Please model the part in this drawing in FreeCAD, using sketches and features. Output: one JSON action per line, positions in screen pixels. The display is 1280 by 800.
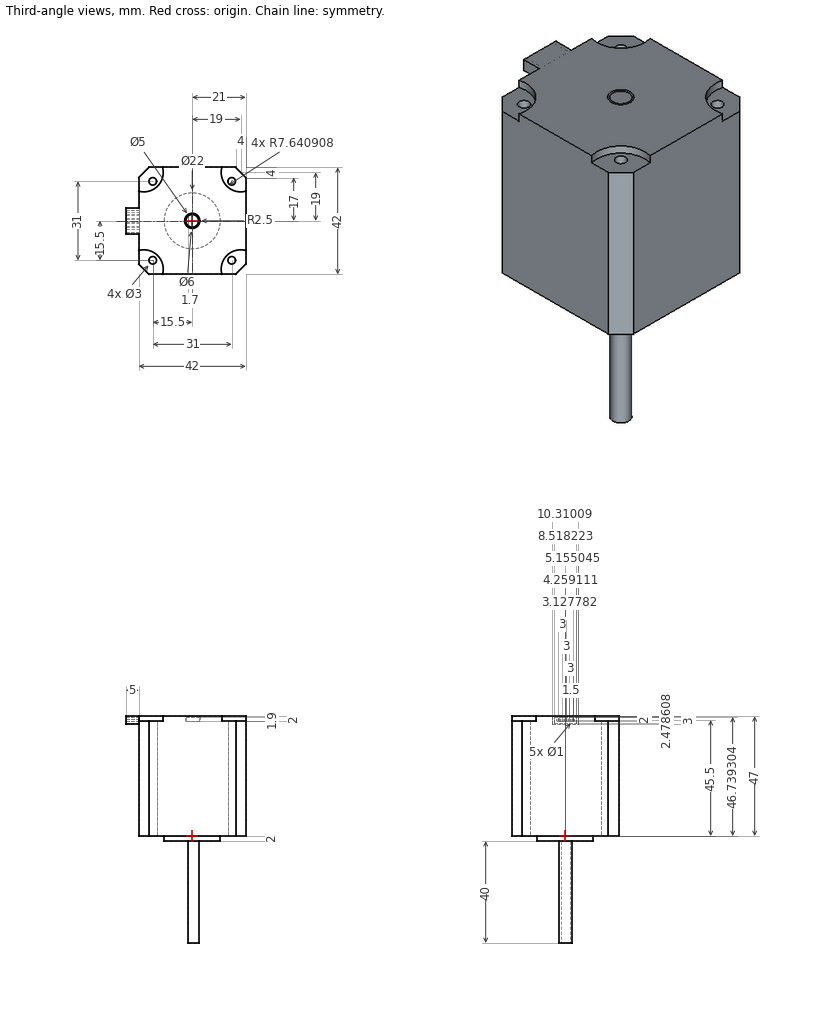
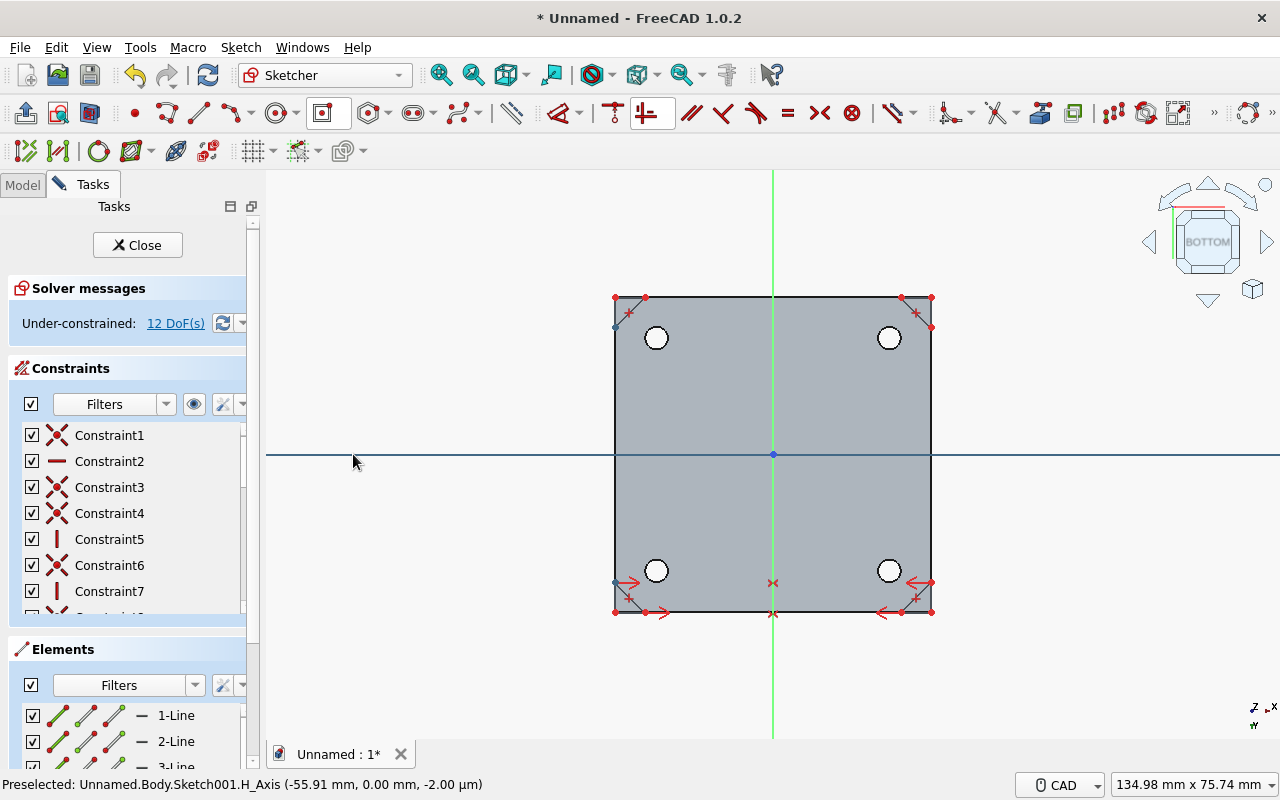
{"action": "left_click", "coordinate": [820, 114]}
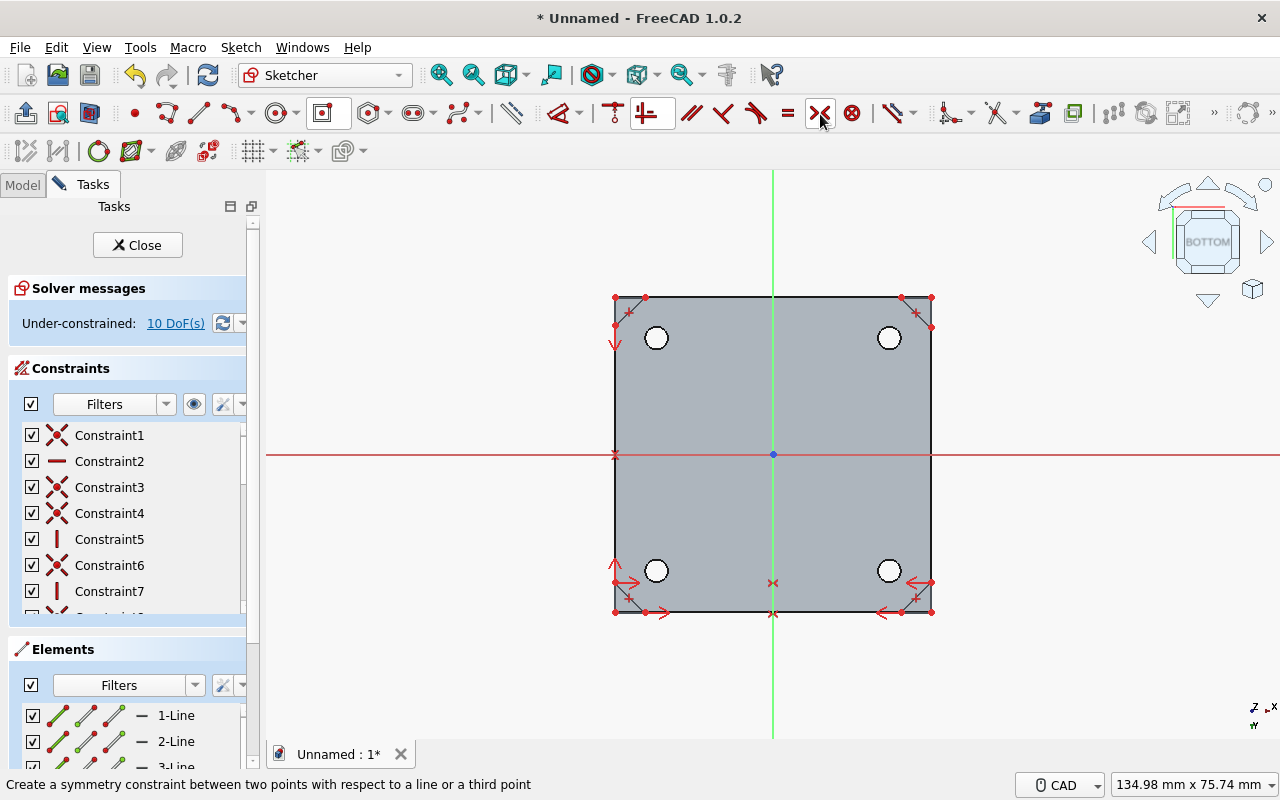
{"action": "left_click", "coordinate": [645, 613]}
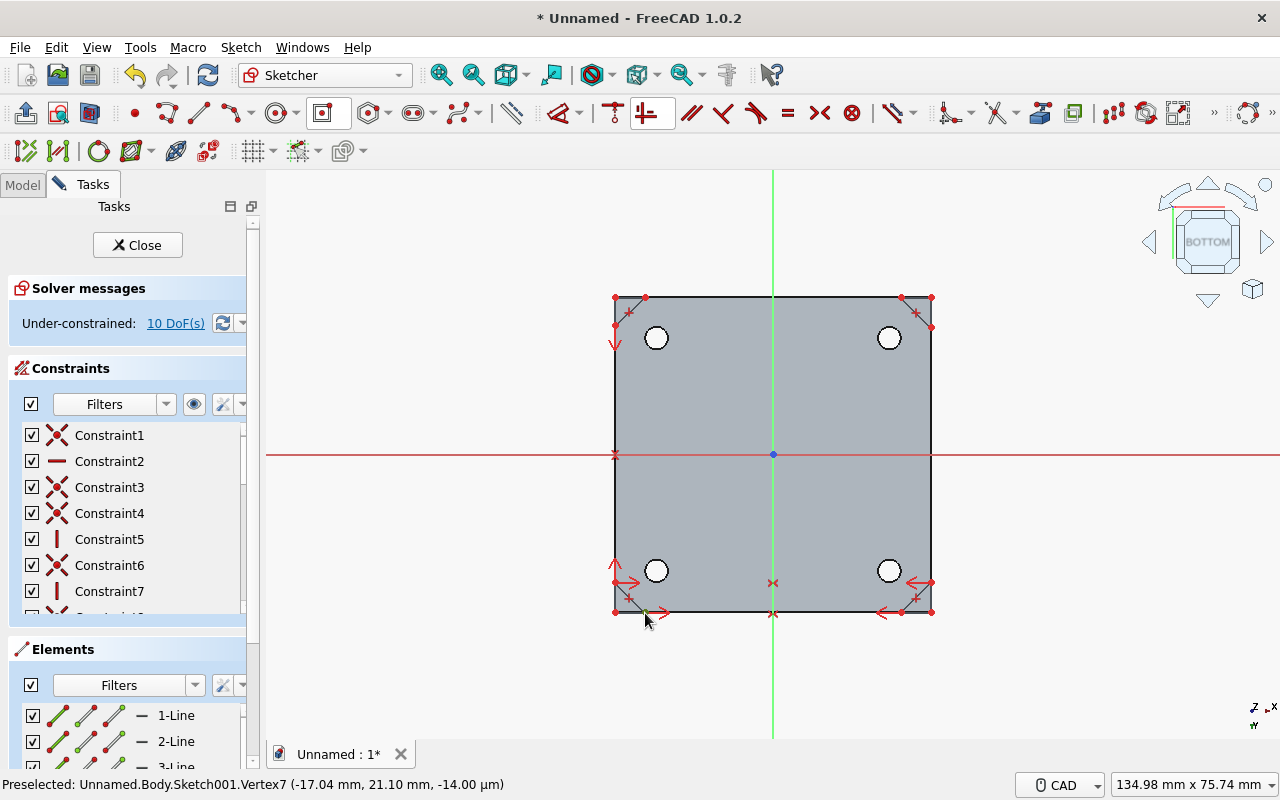
{"action": "left_click", "coordinate": [645, 298]}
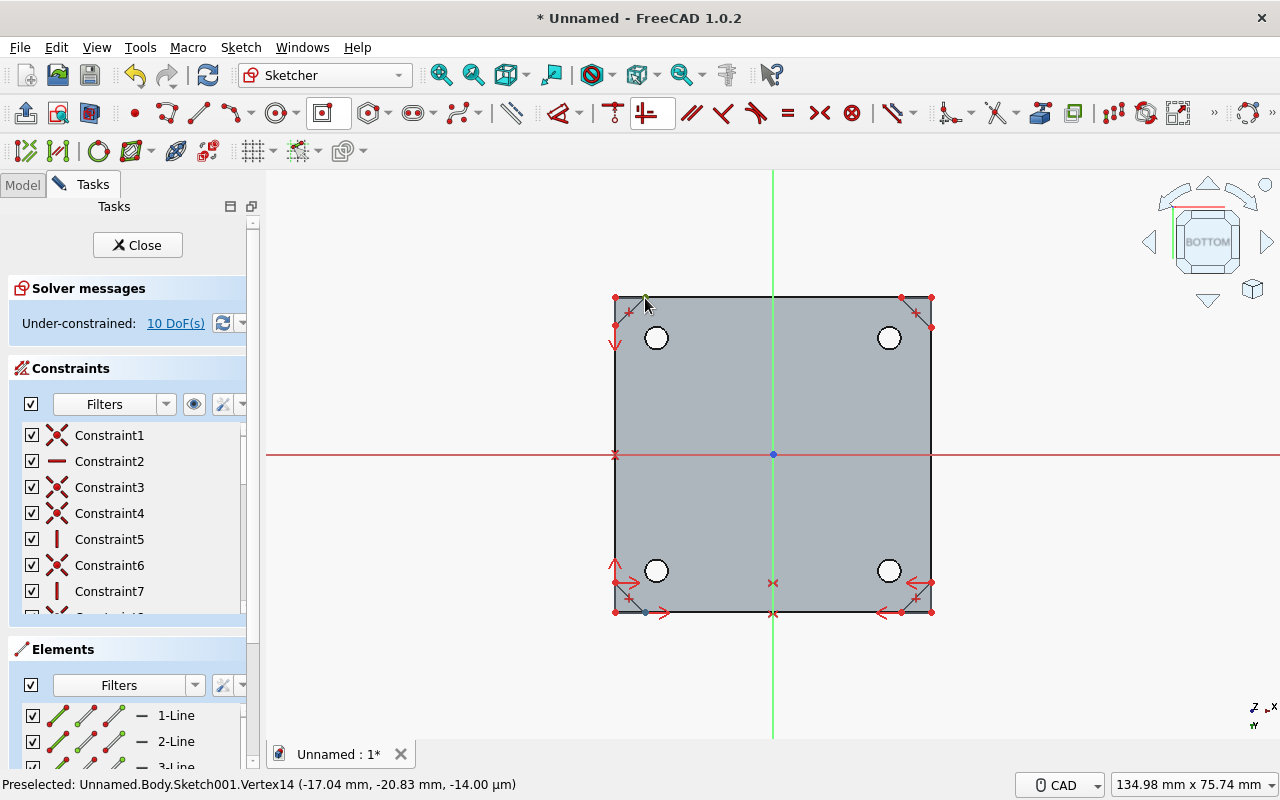
{"action": "left_click", "coordinate": [353, 454]}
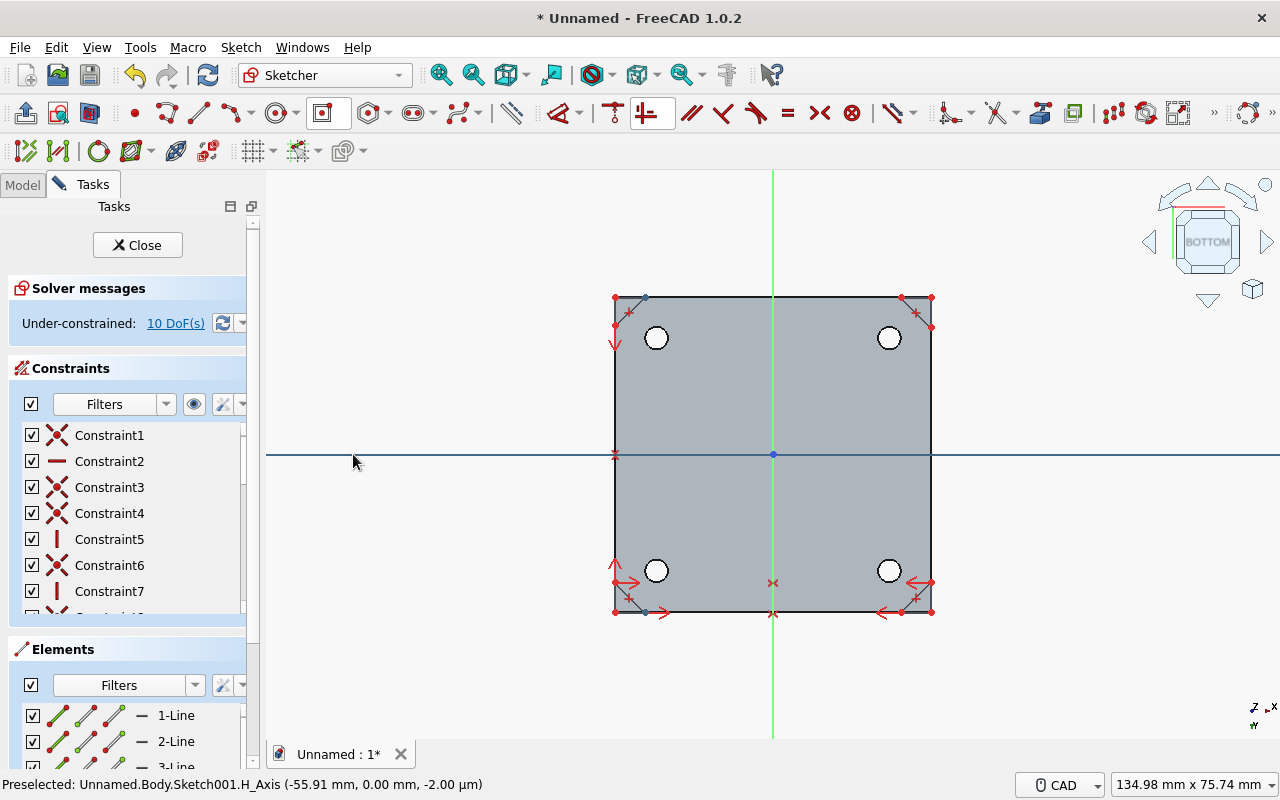
{"action": "left_click", "coordinate": [820, 114]}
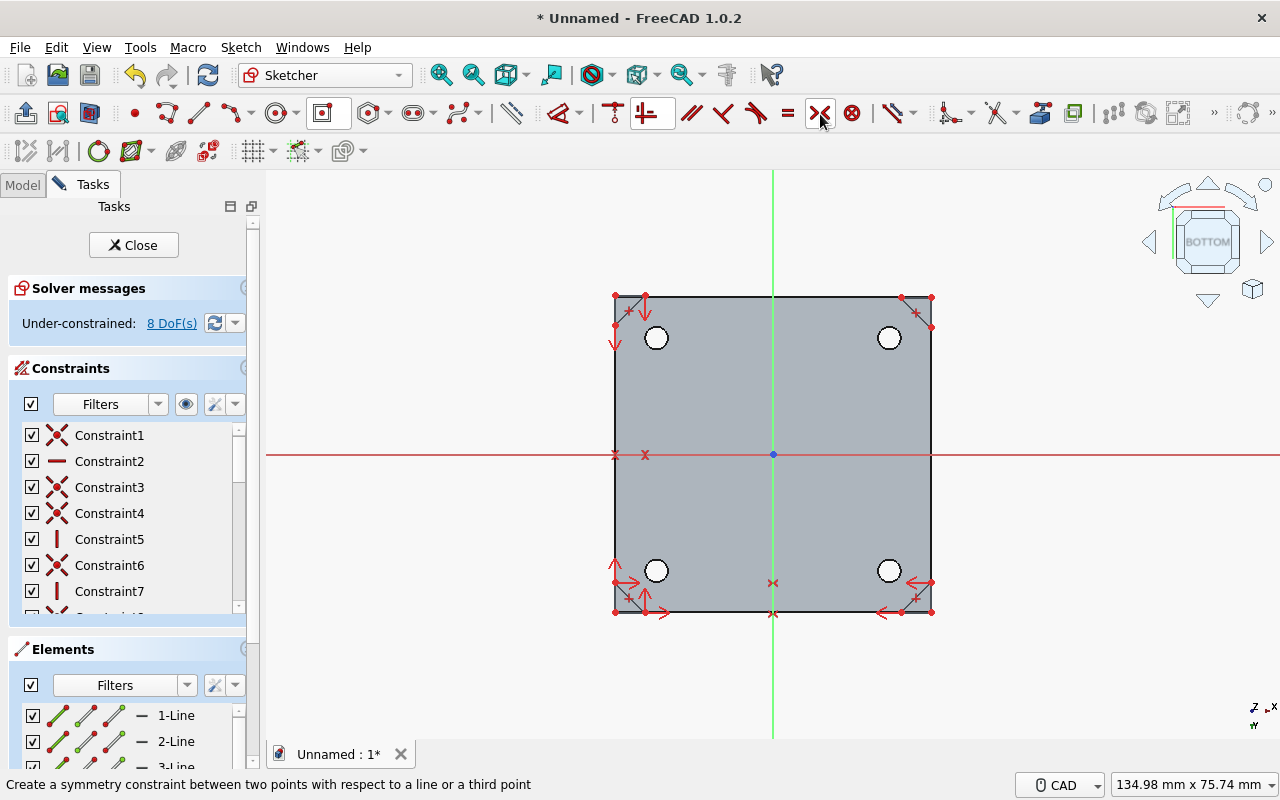
{"action": "left_click", "coordinate": [901, 613]}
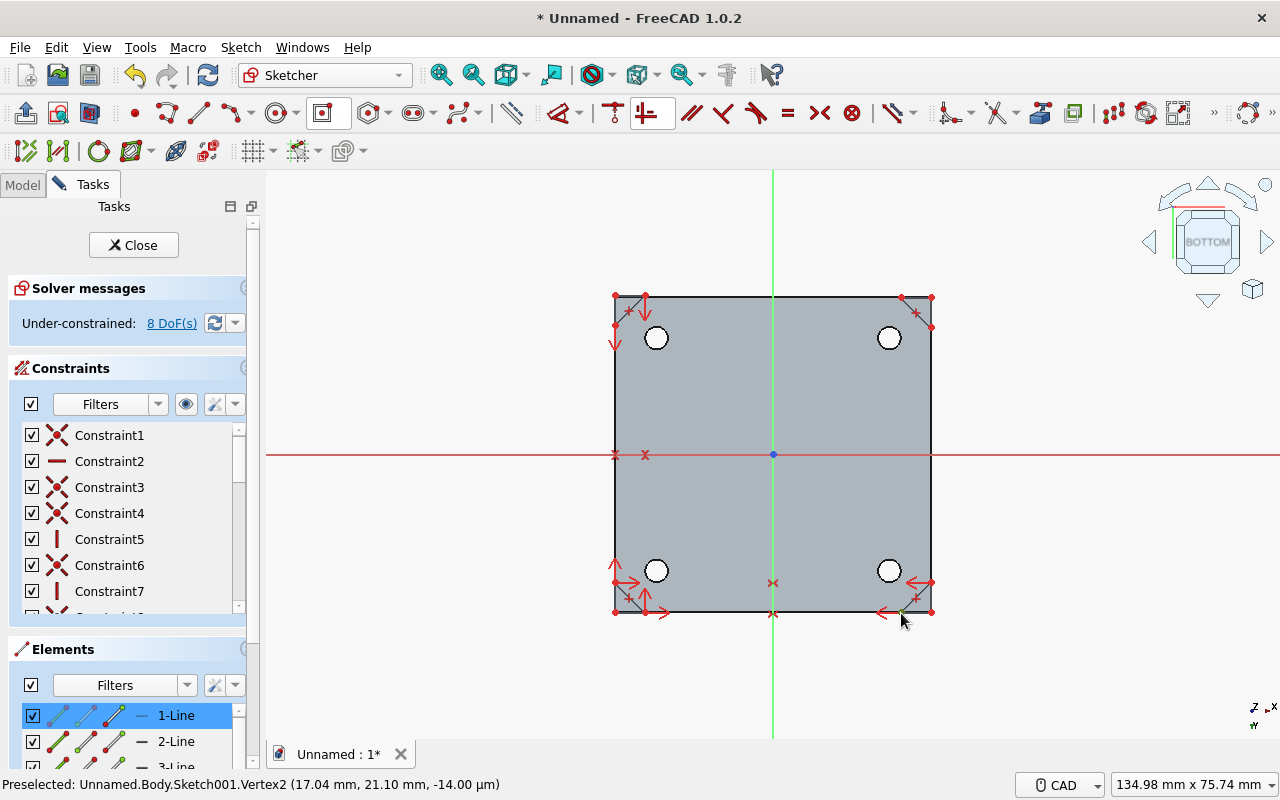
{"action": "left_click", "coordinate": [901, 298]}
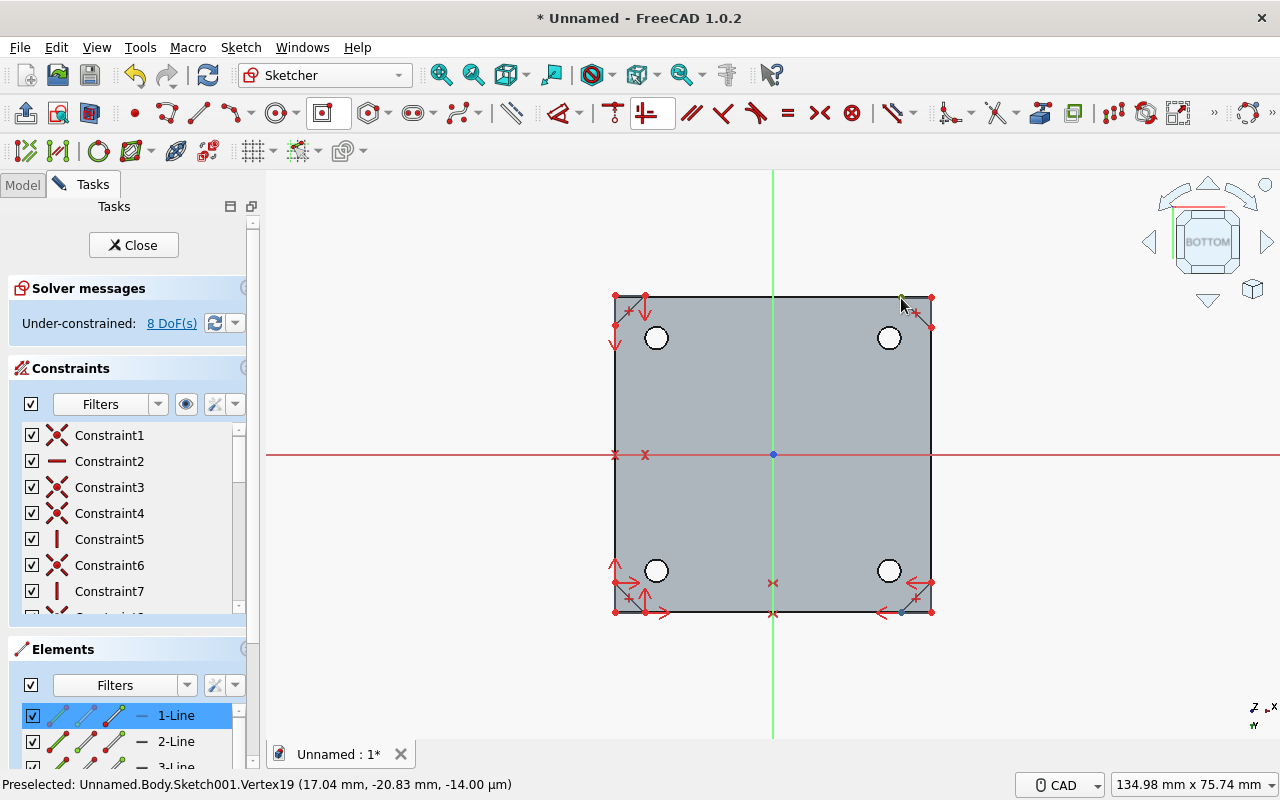
{"action": "left_click", "coordinate": [353, 454]}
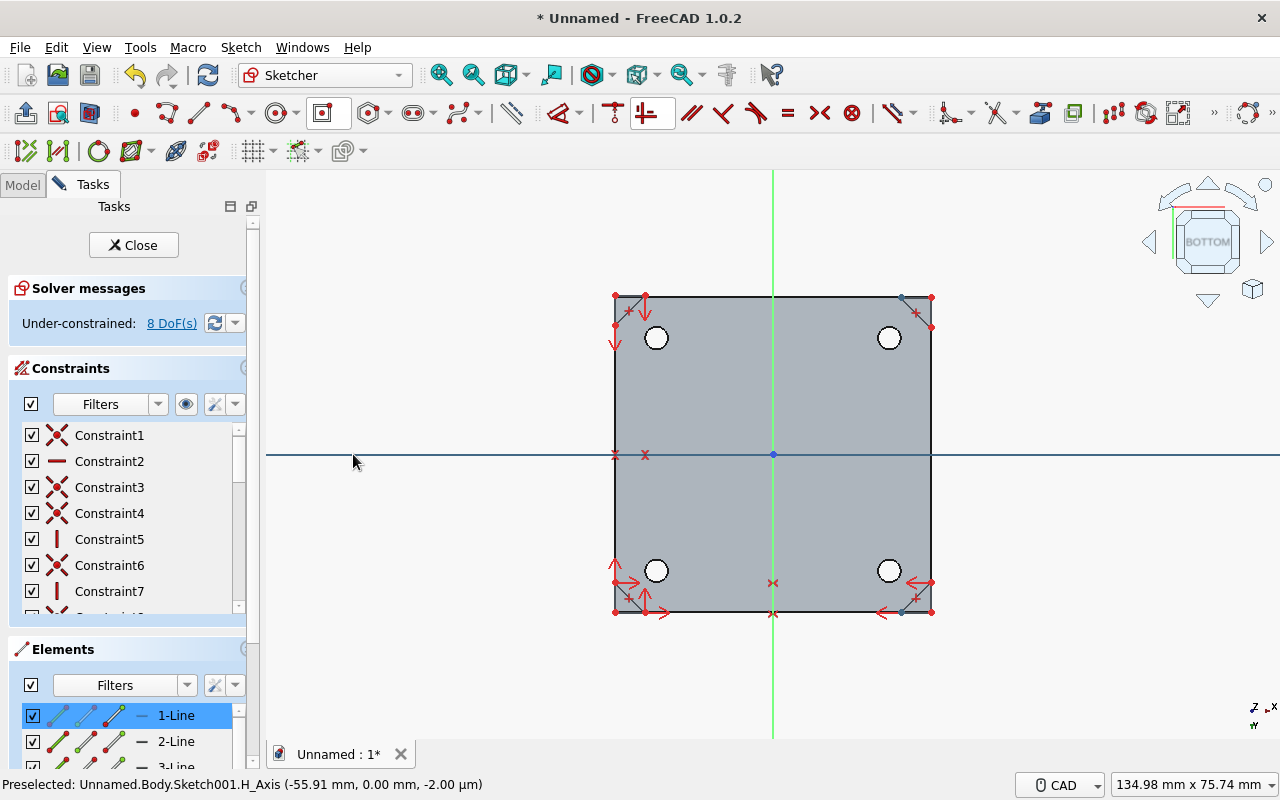
{"action": "left_click", "coordinate": [820, 114]}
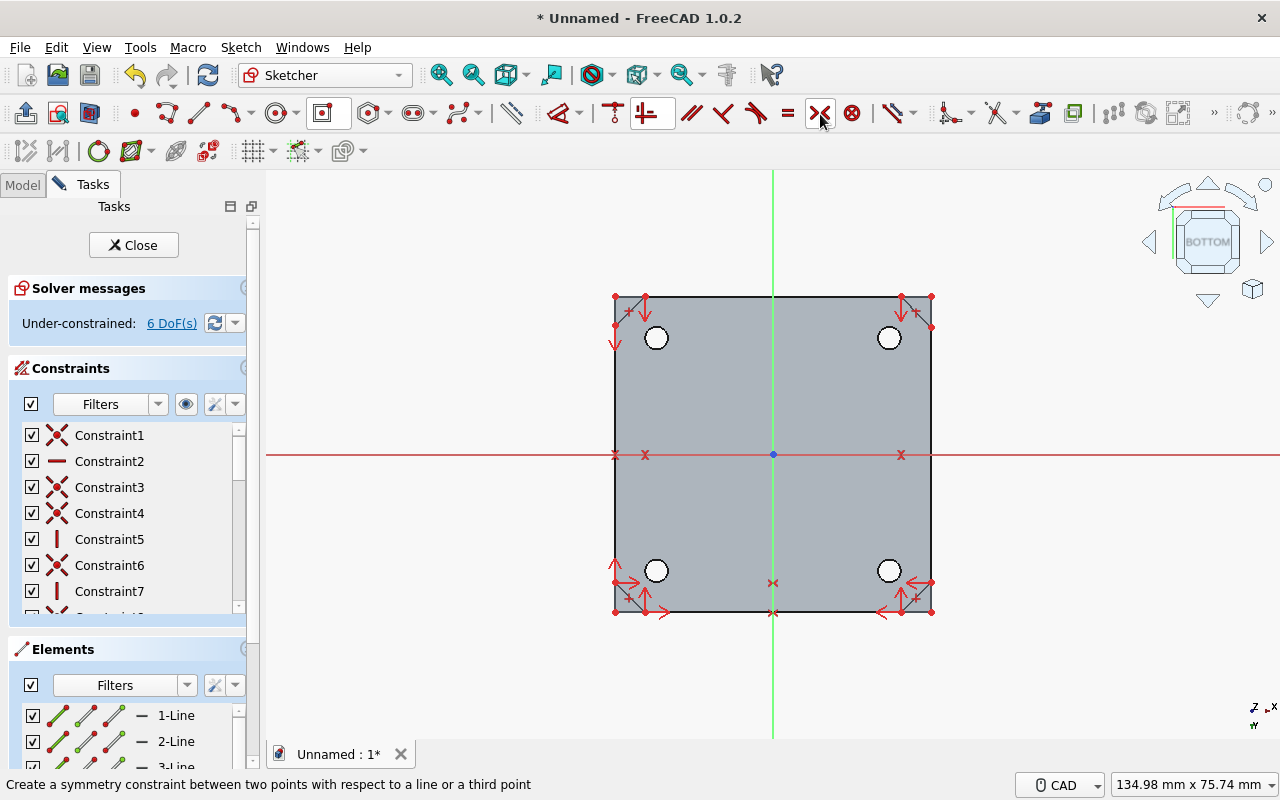
{"action": "left_click", "coordinate": [931, 583]}